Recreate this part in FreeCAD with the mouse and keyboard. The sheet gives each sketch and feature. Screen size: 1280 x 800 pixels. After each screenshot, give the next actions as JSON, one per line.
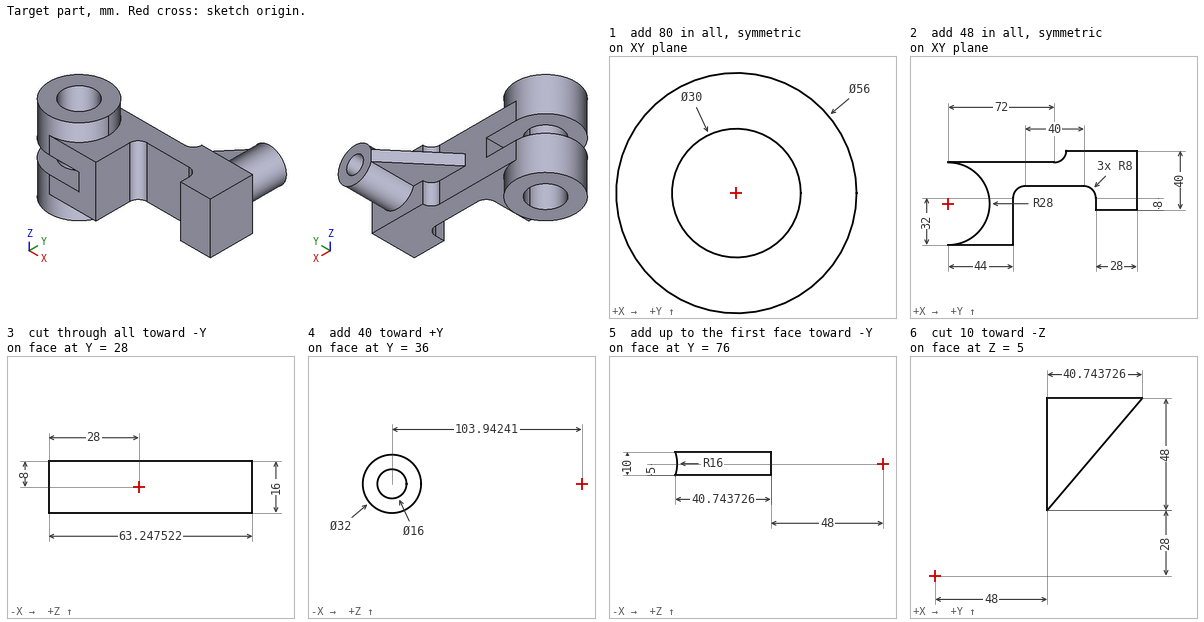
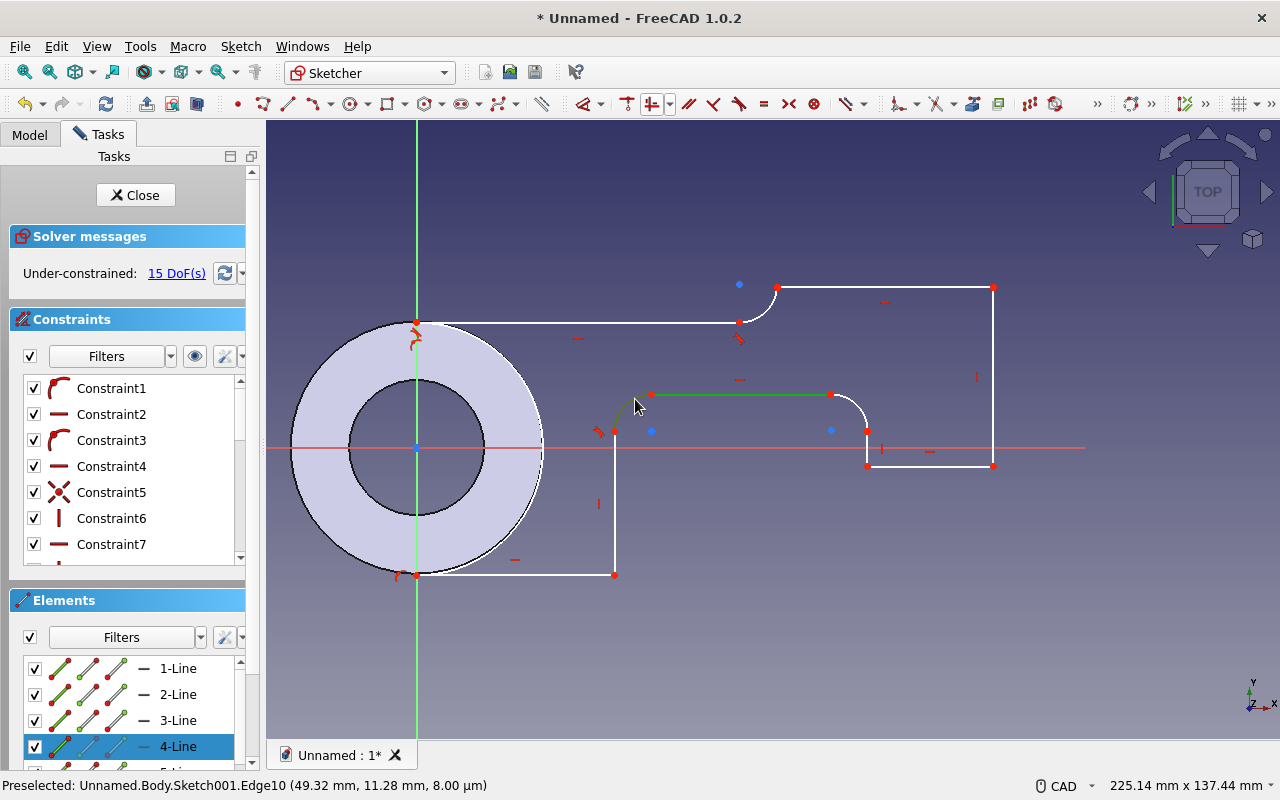
{"action": "left_click", "coordinate": [739, 104]}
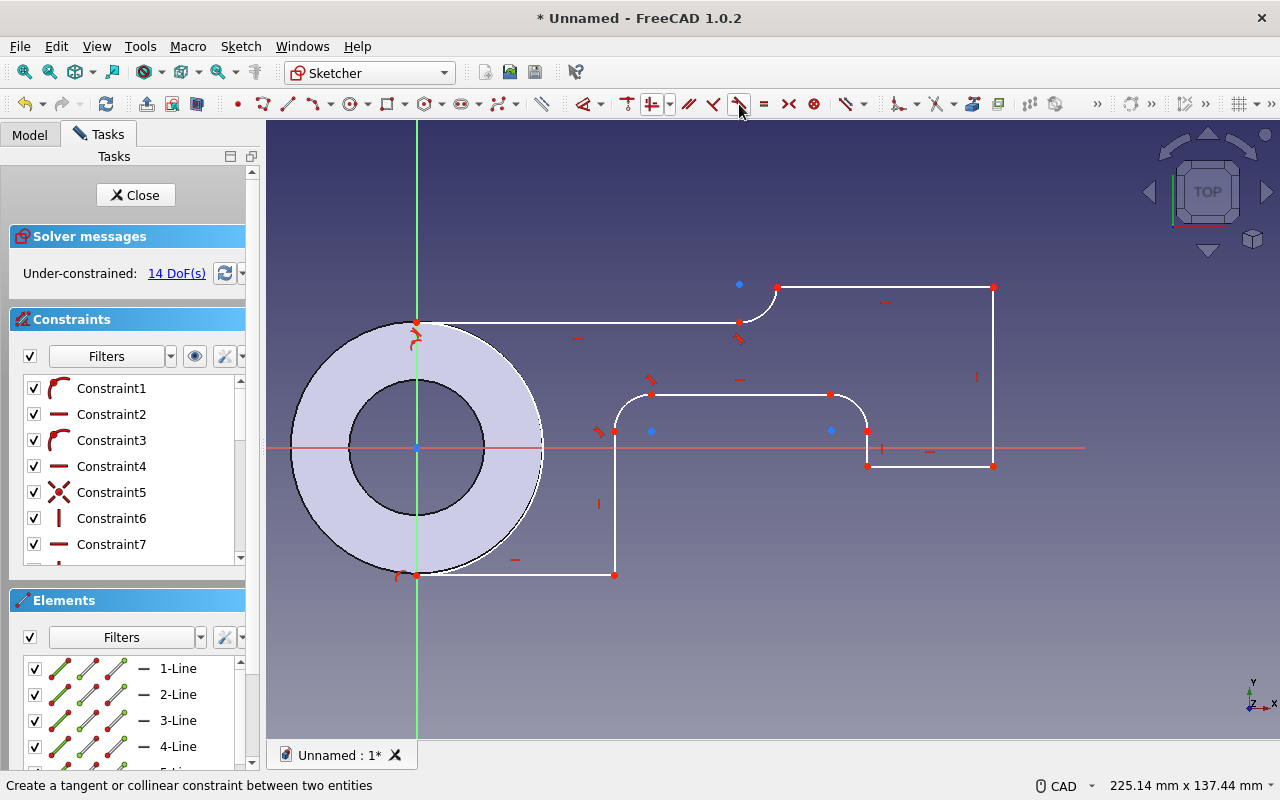
{"action": "left_click", "coordinate": [705, 395]}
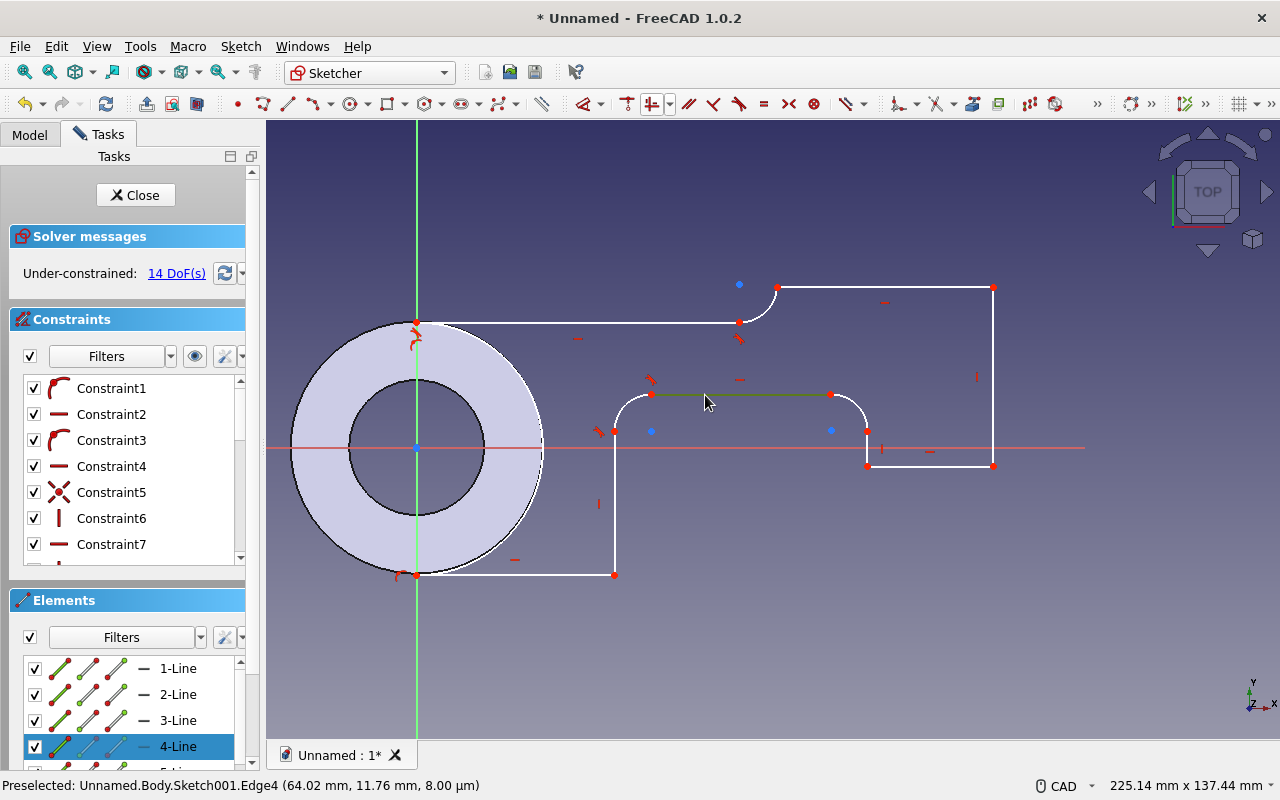
{"action": "left_click", "coordinate": [864, 414]}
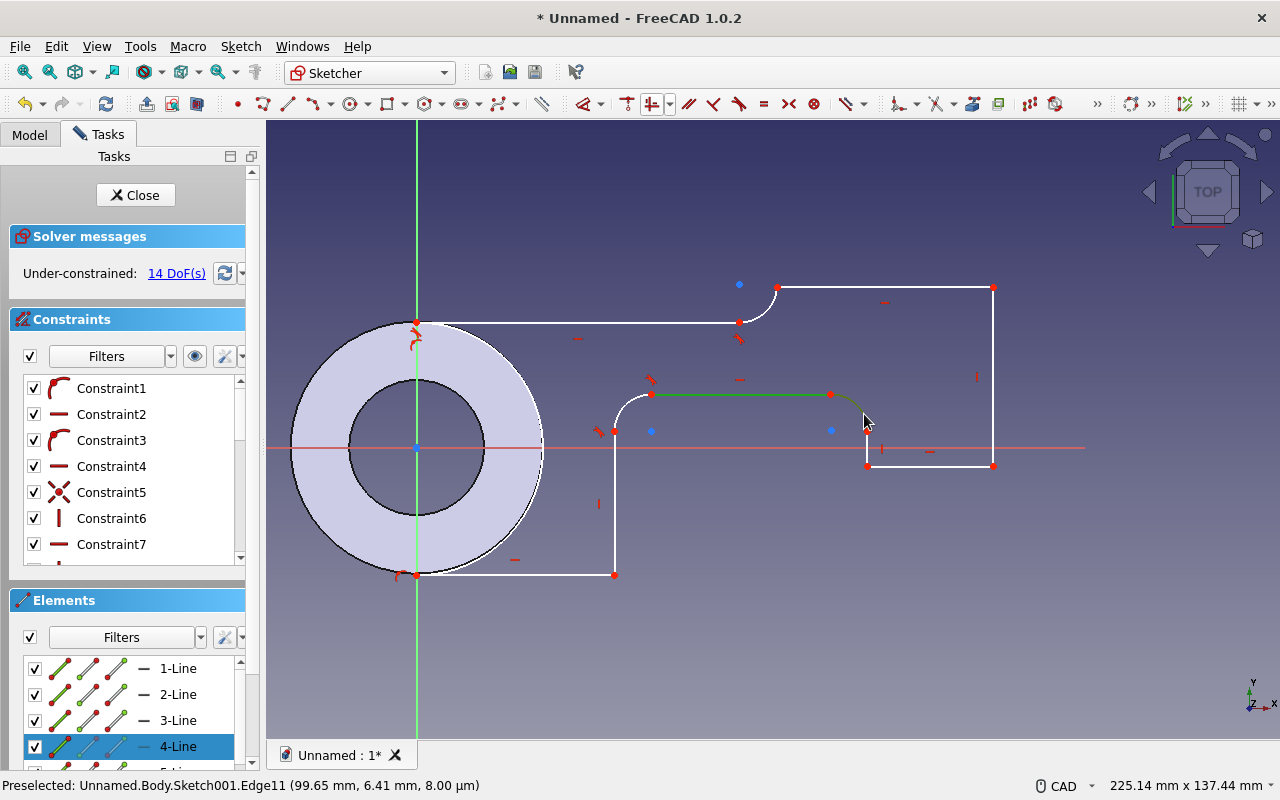
{"action": "left_click", "coordinate": [739, 104]}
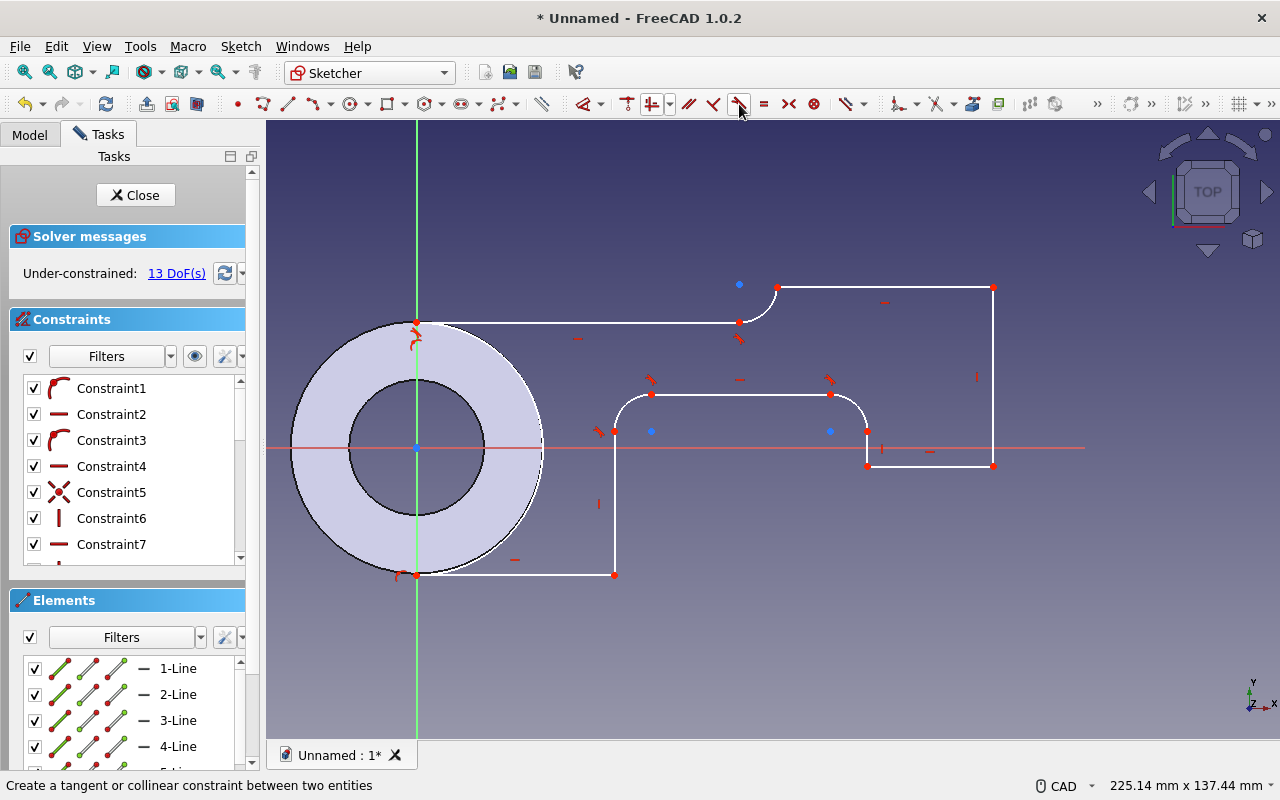
{"action": "left_click", "coordinate": [867, 445]}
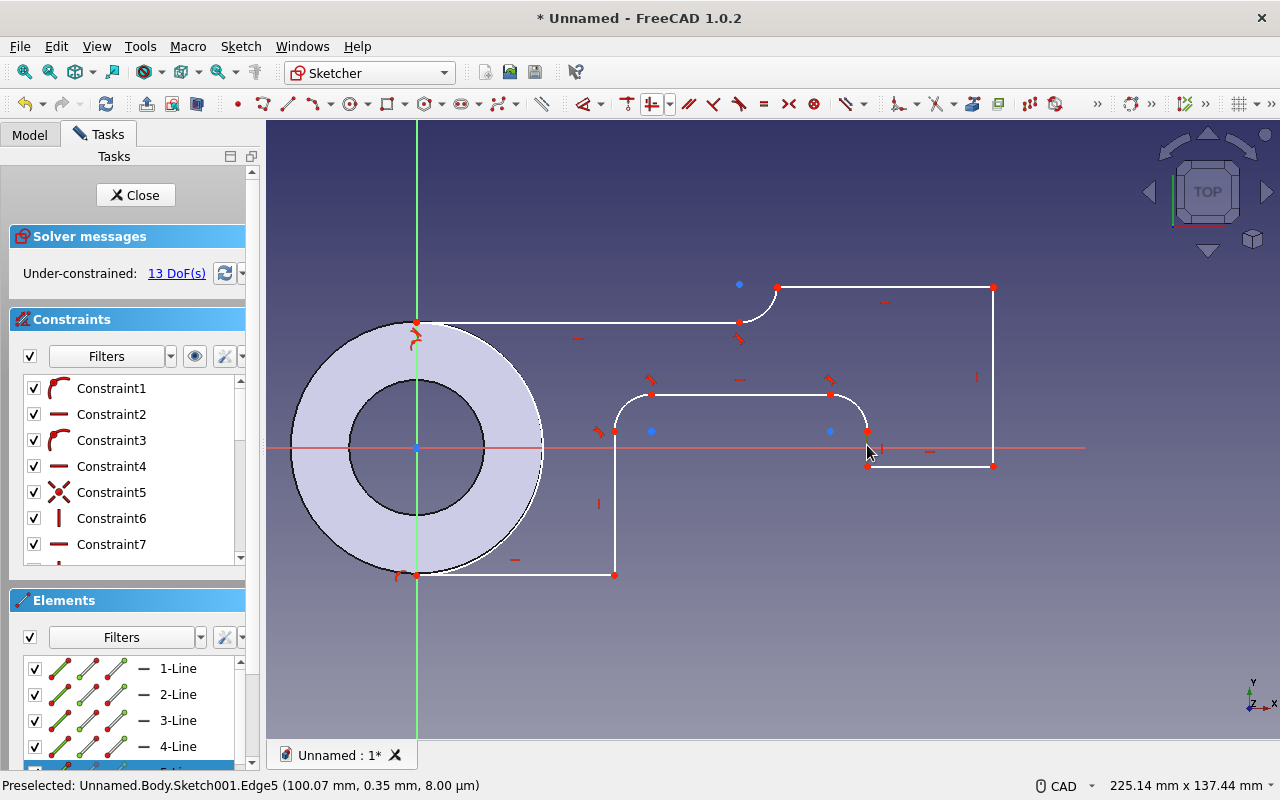
{"action": "left_click", "coordinate": [863, 415]}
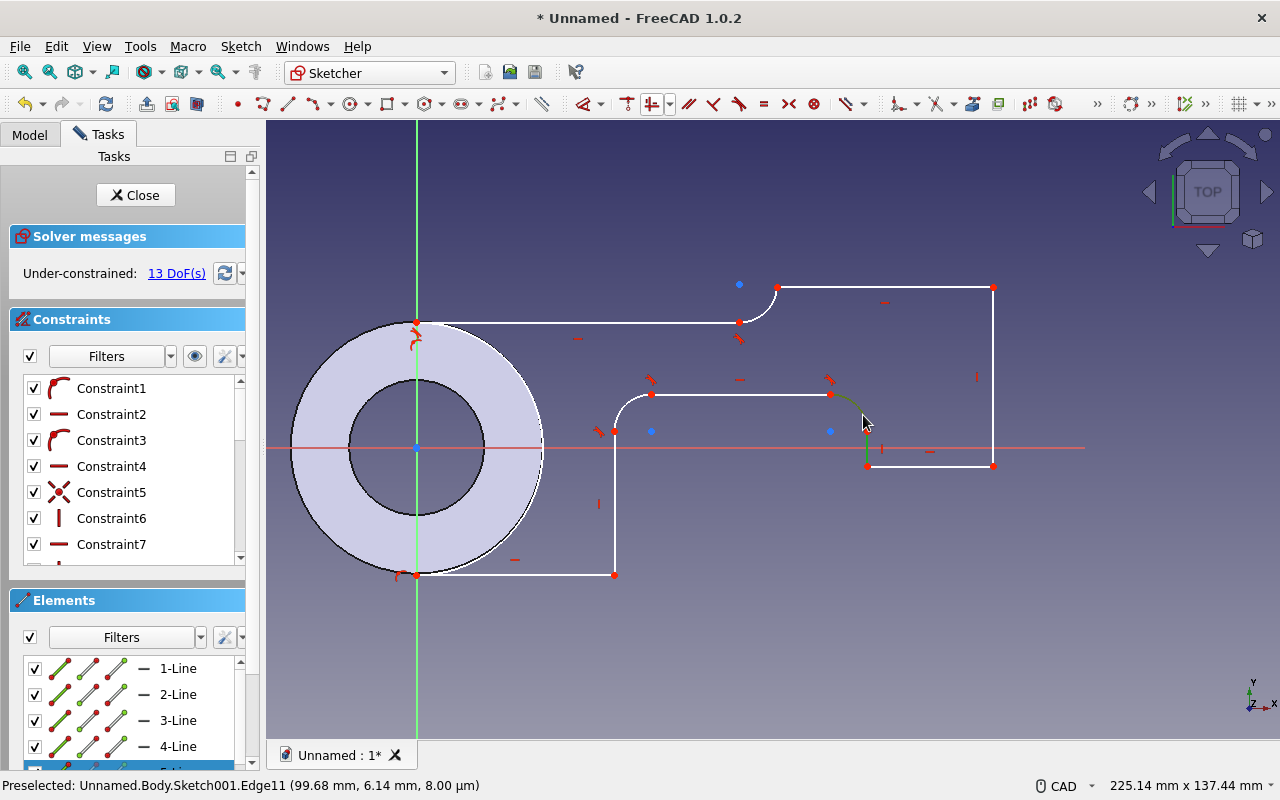
{"action": "left_click", "coordinate": [739, 104]}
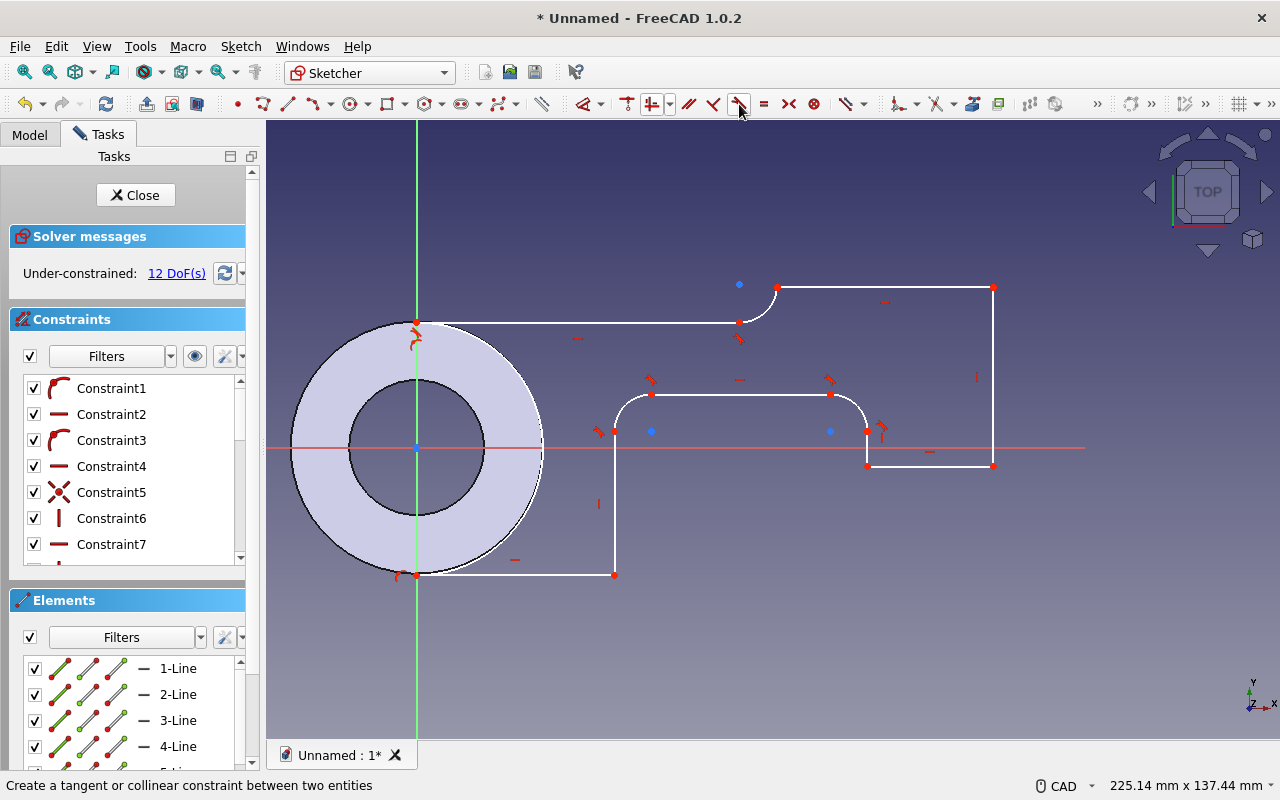
{"action": "left_click", "coordinate": [635, 399]}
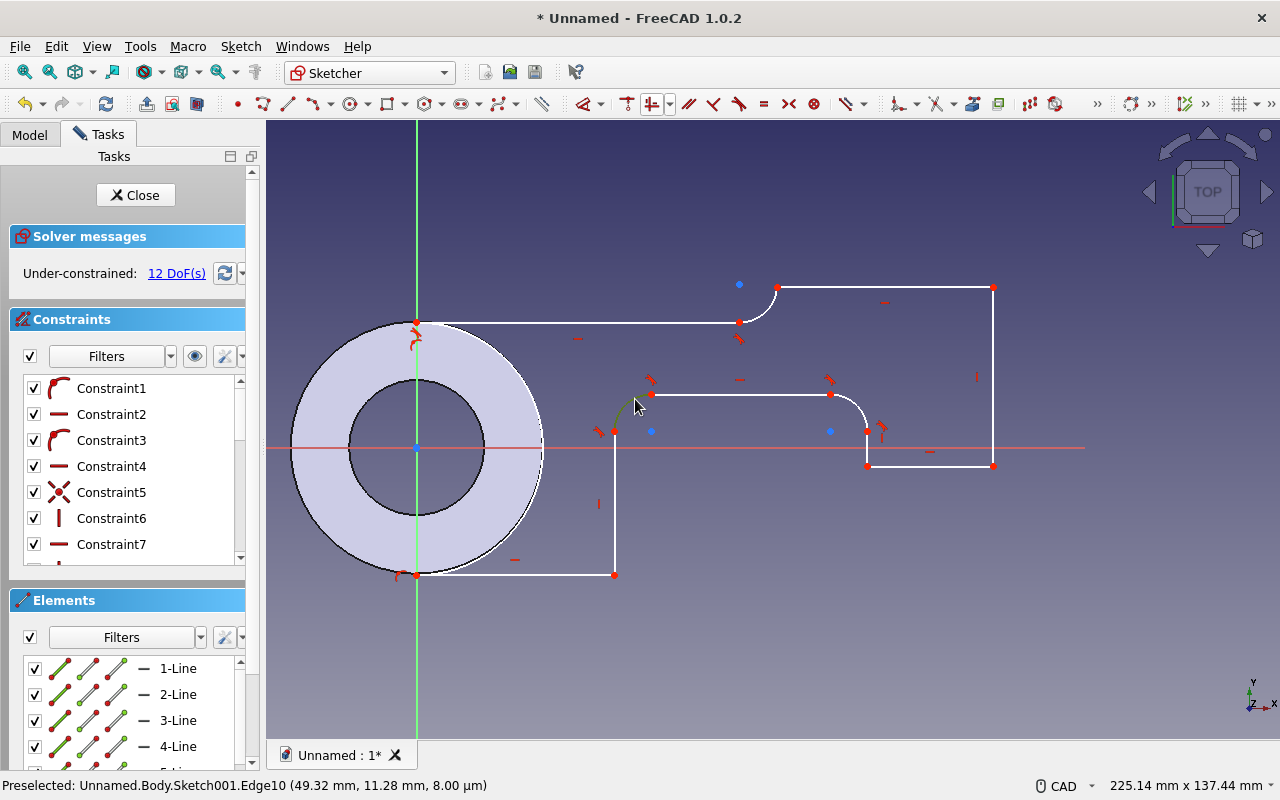
{"action": "left_click", "coordinate": [863, 415]}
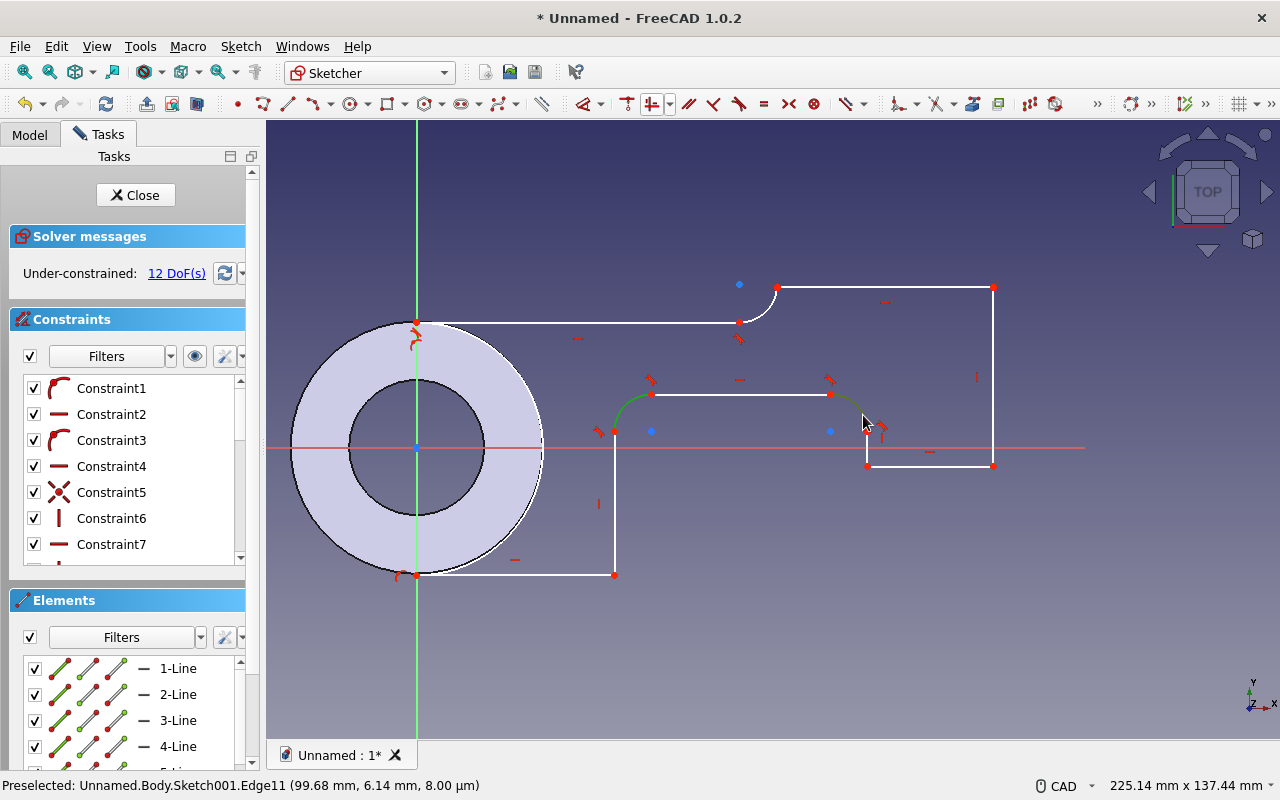
{"action": "left_click", "coordinate": [756, 319]}